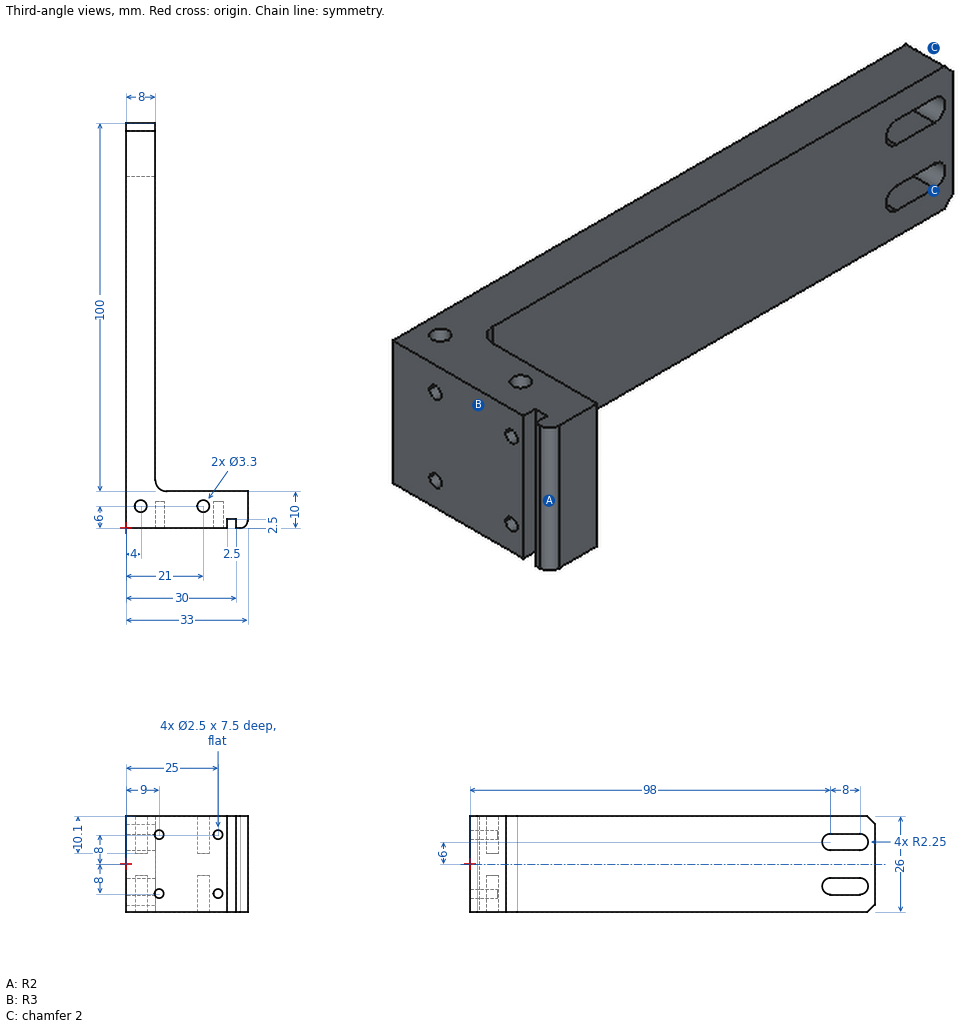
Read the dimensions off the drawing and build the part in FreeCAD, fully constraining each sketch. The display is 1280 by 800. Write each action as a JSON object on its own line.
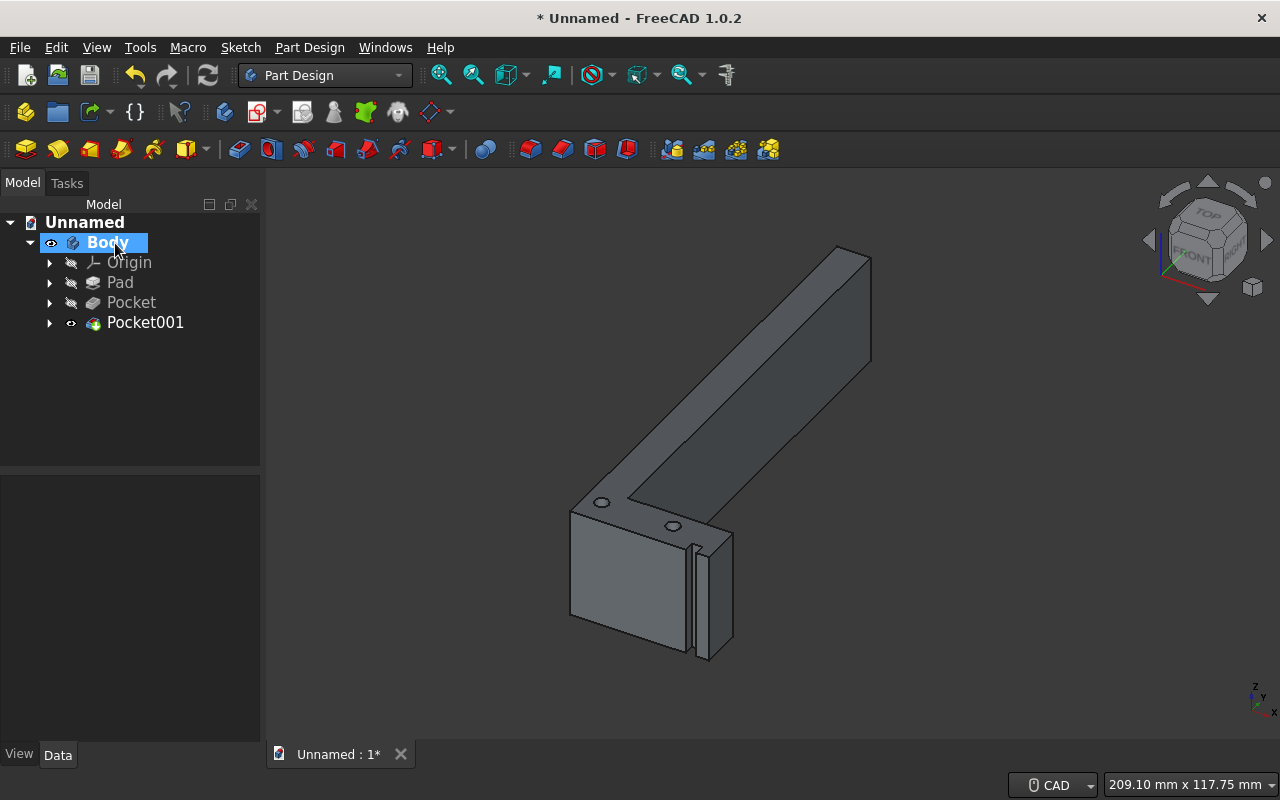
{"action": "left_click", "coordinate": [116, 323]}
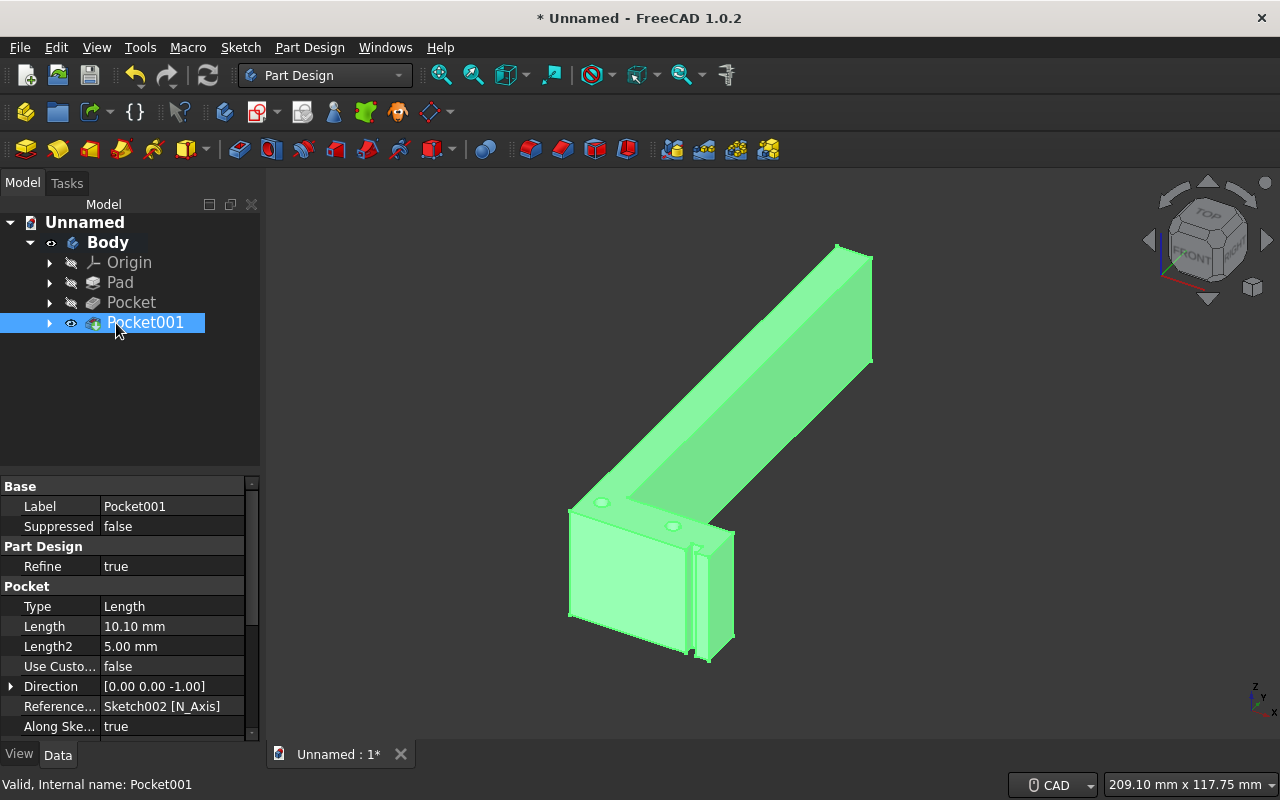
{"action": "left_click", "coordinate": [672, 150]}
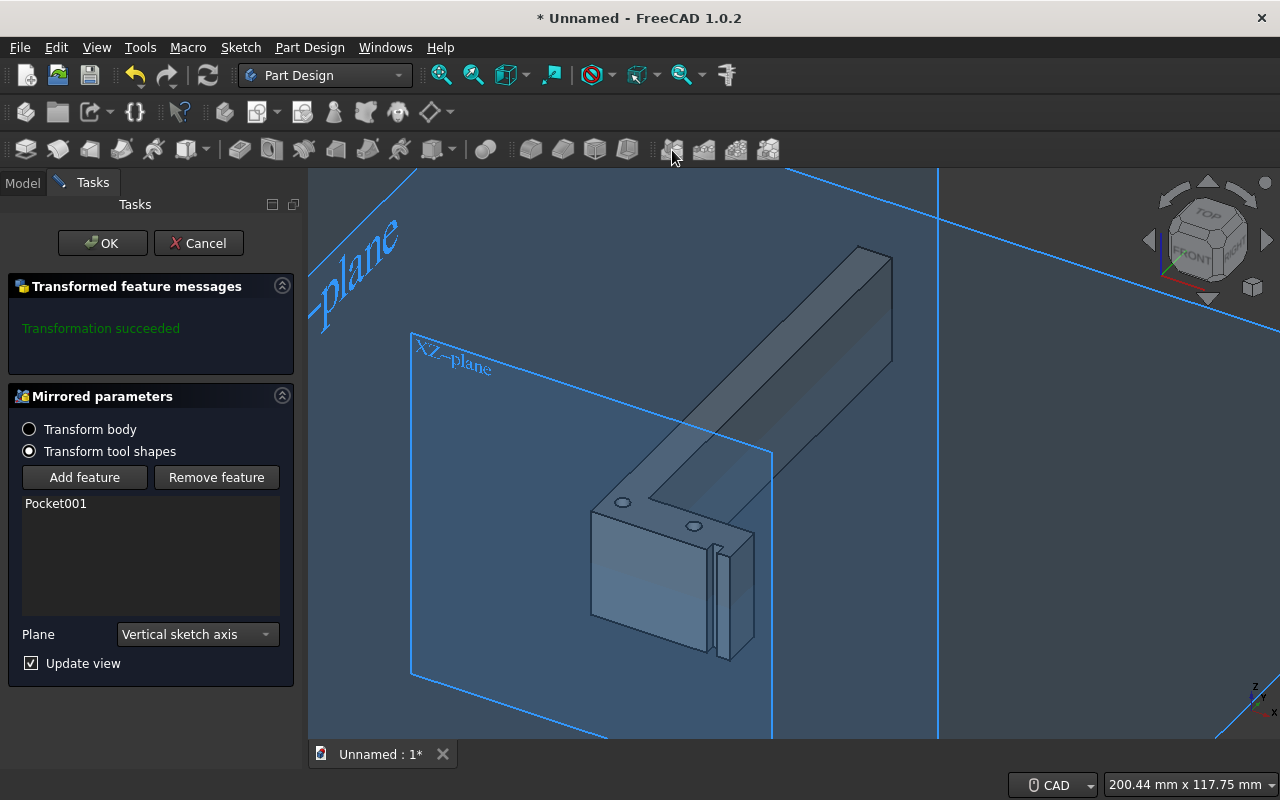
{"action": "left_click", "coordinate": [198, 634]}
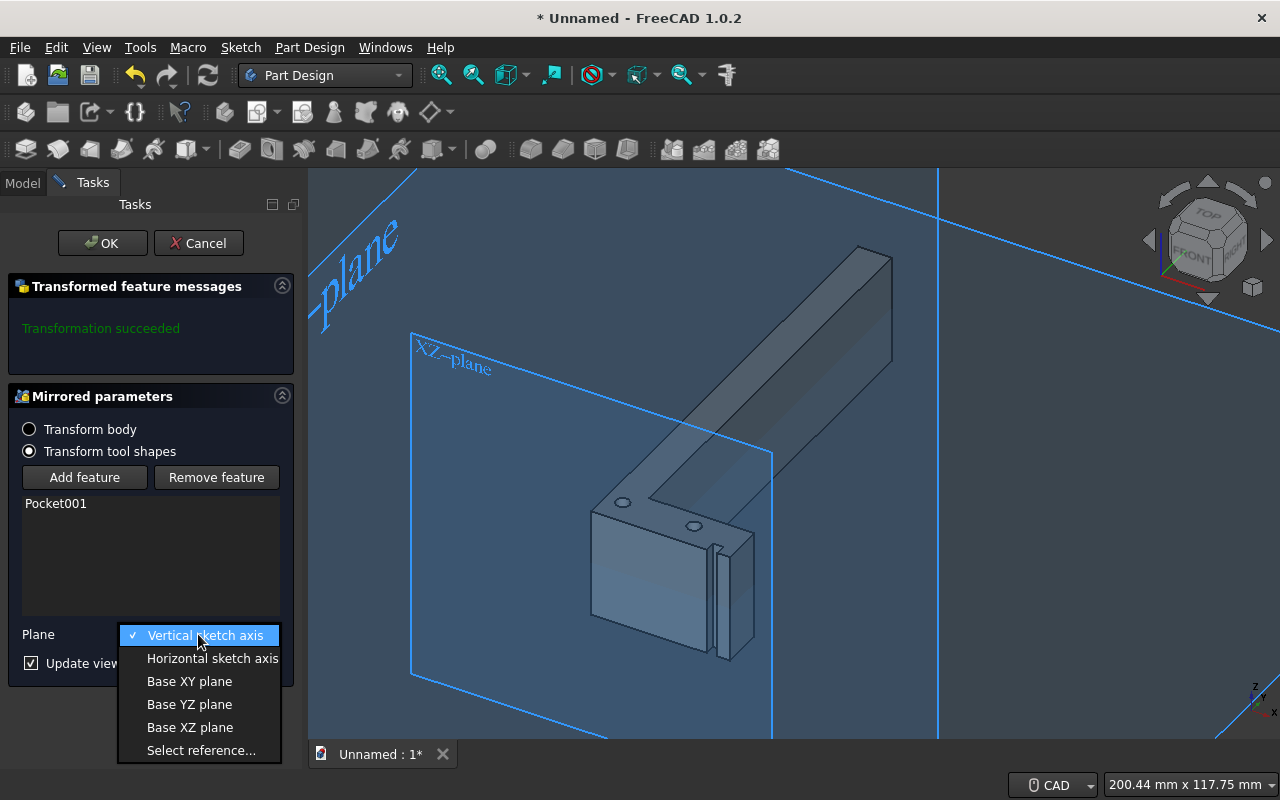
{"action": "left_click", "coordinate": [198, 682]}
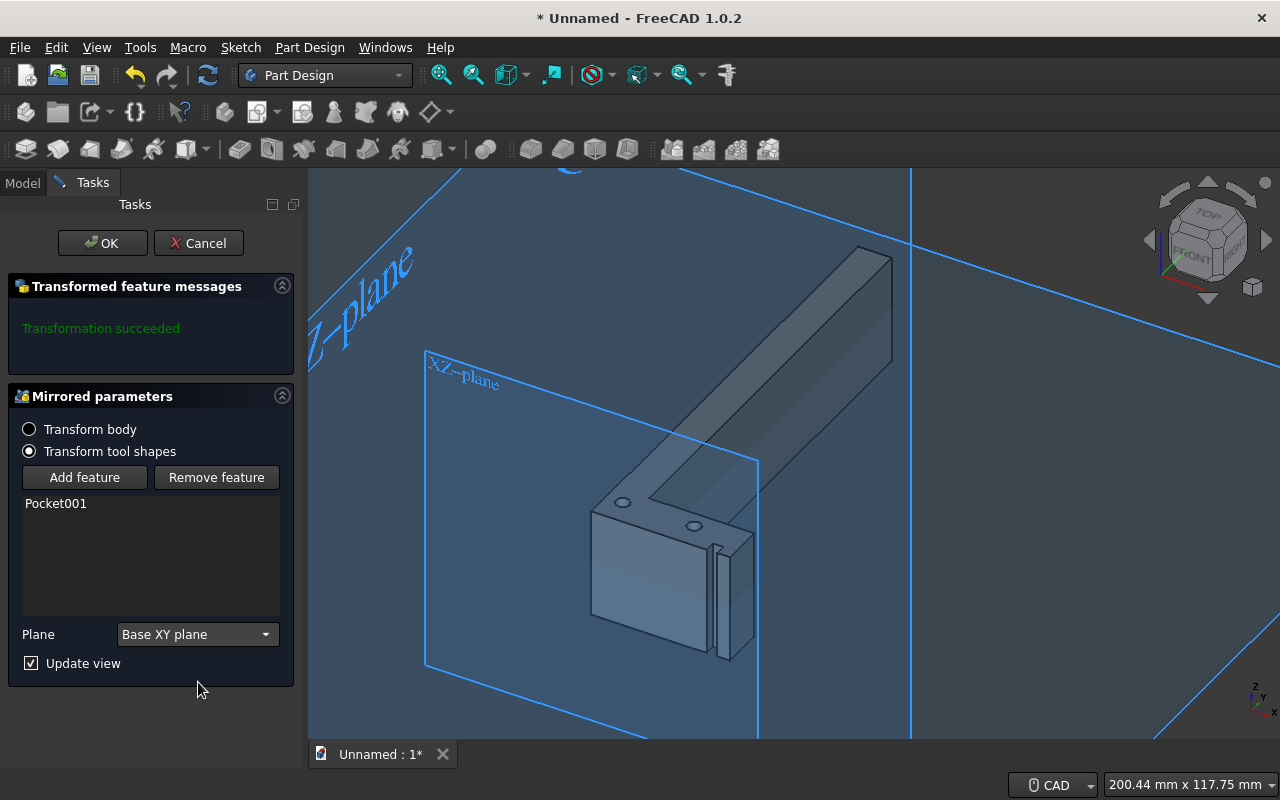
{"action": "left_click", "coordinate": [103, 243]}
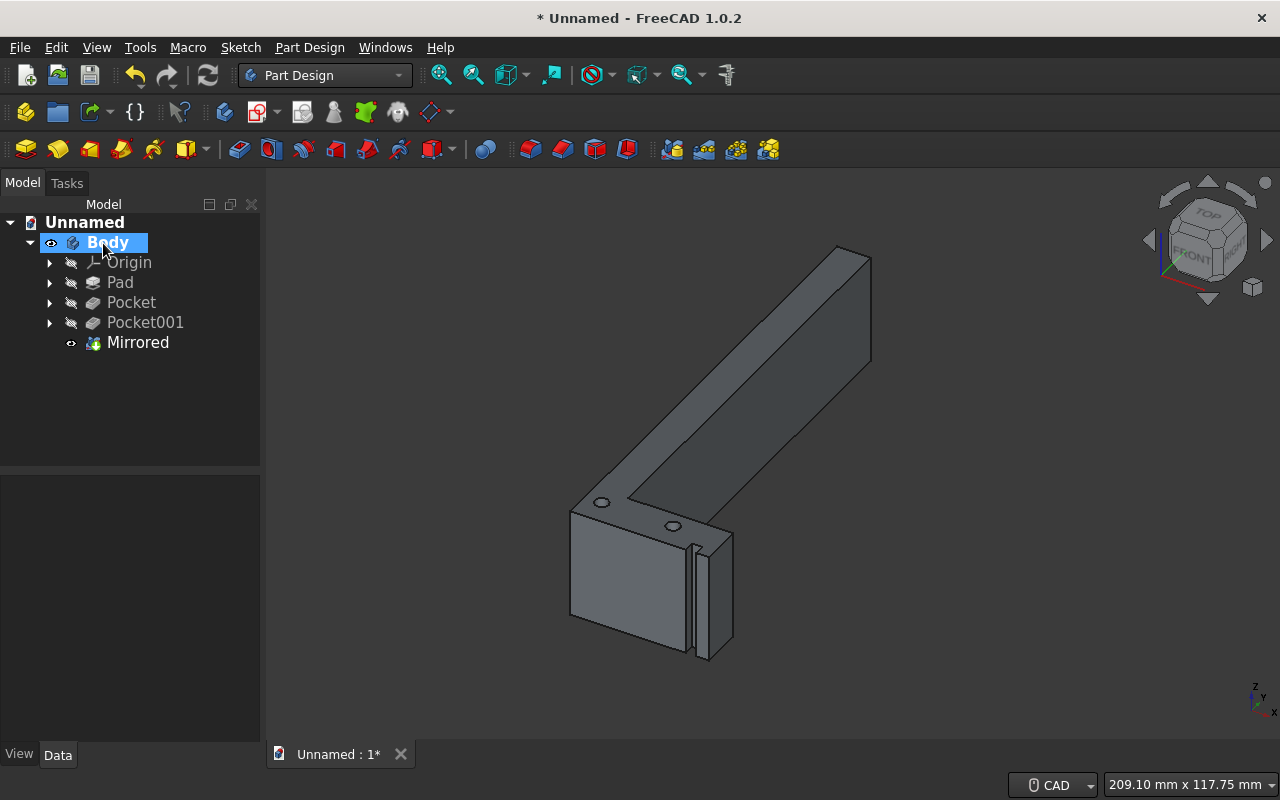
{"action": "left_click", "coordinate": [258, 112]}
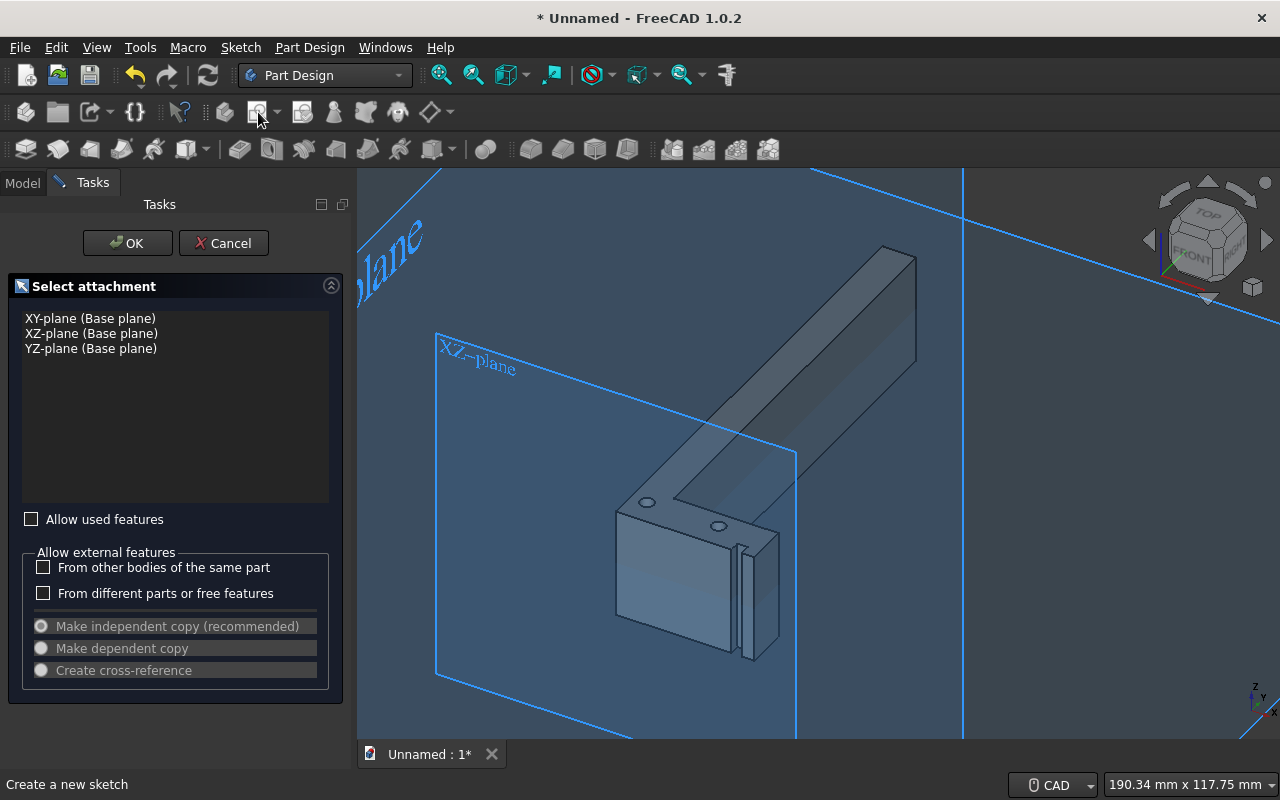
{"action": "left_click", "coordinate": [82, 334]}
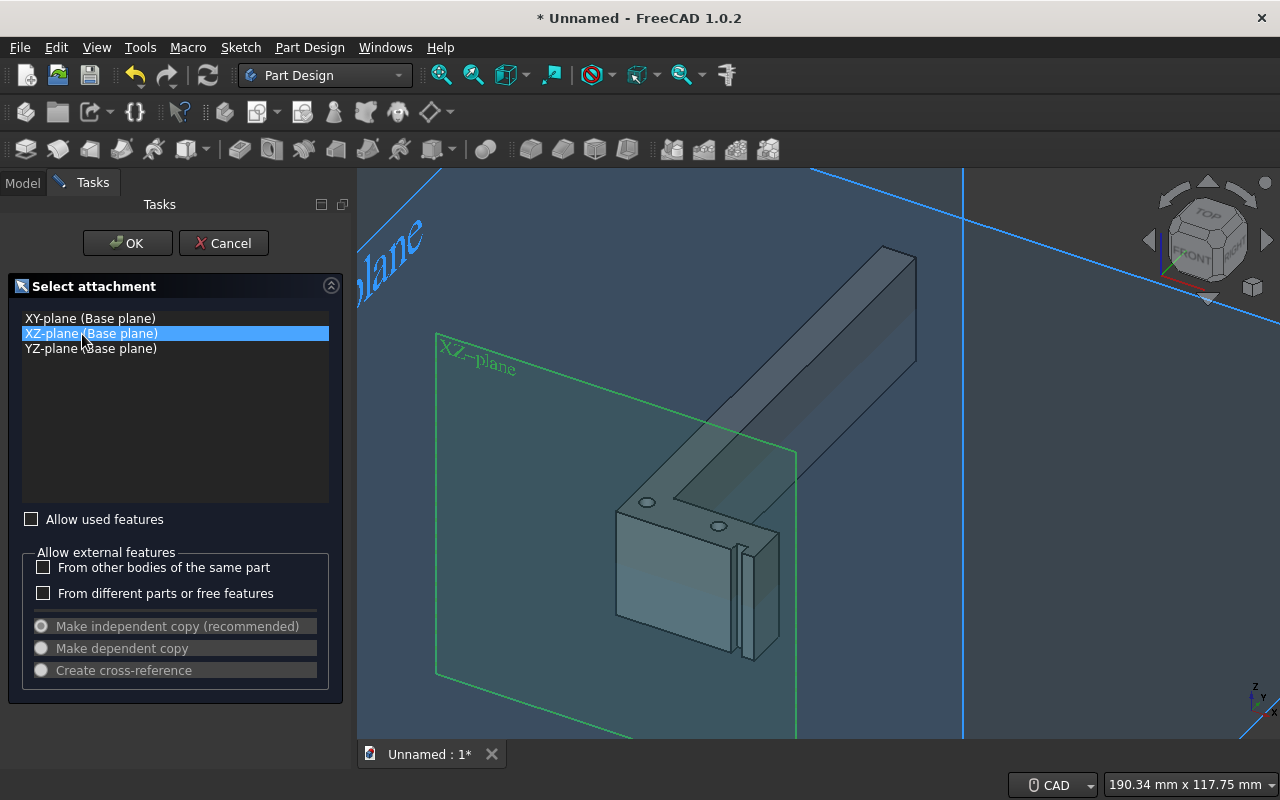
{"action": "left_click", "coordinate": [128, 243]}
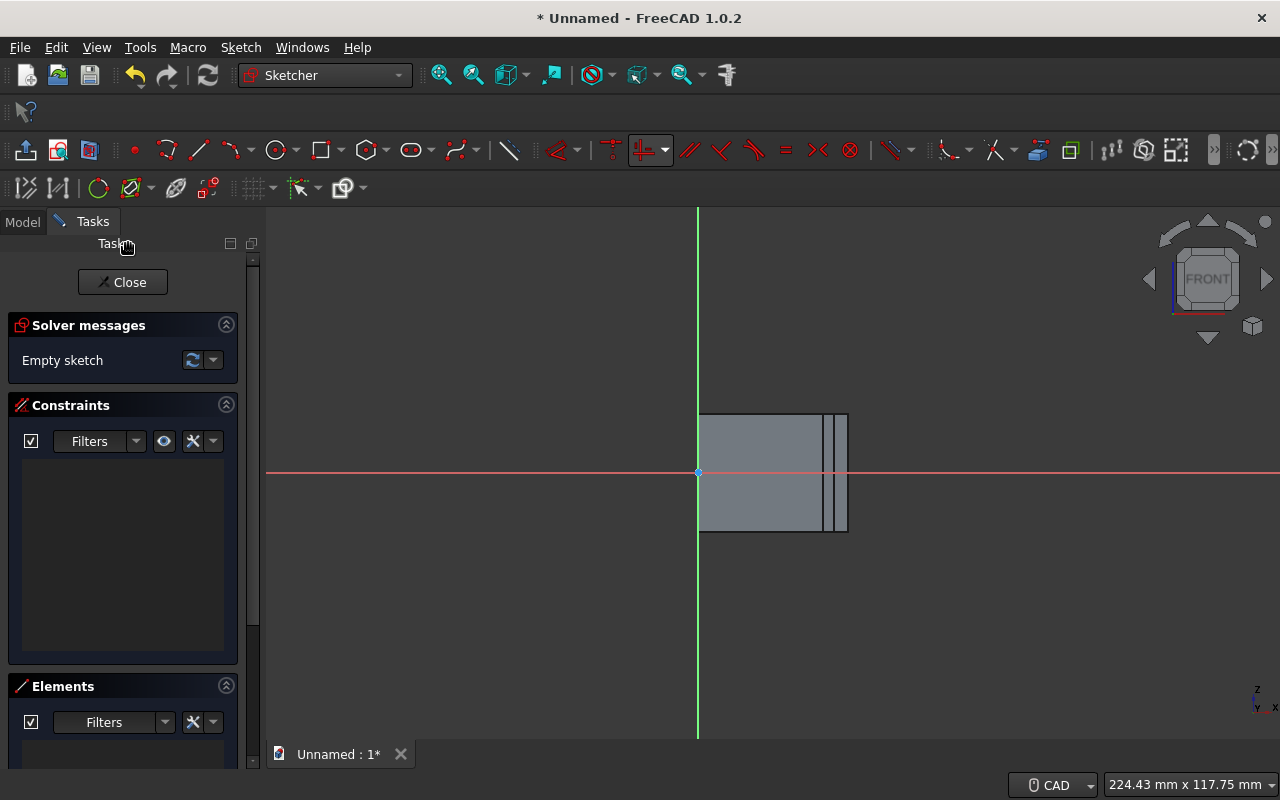
{"action": "scroll", "coordinate": [775, 473], "scroll_direction": "up", "scroll_amount": 7}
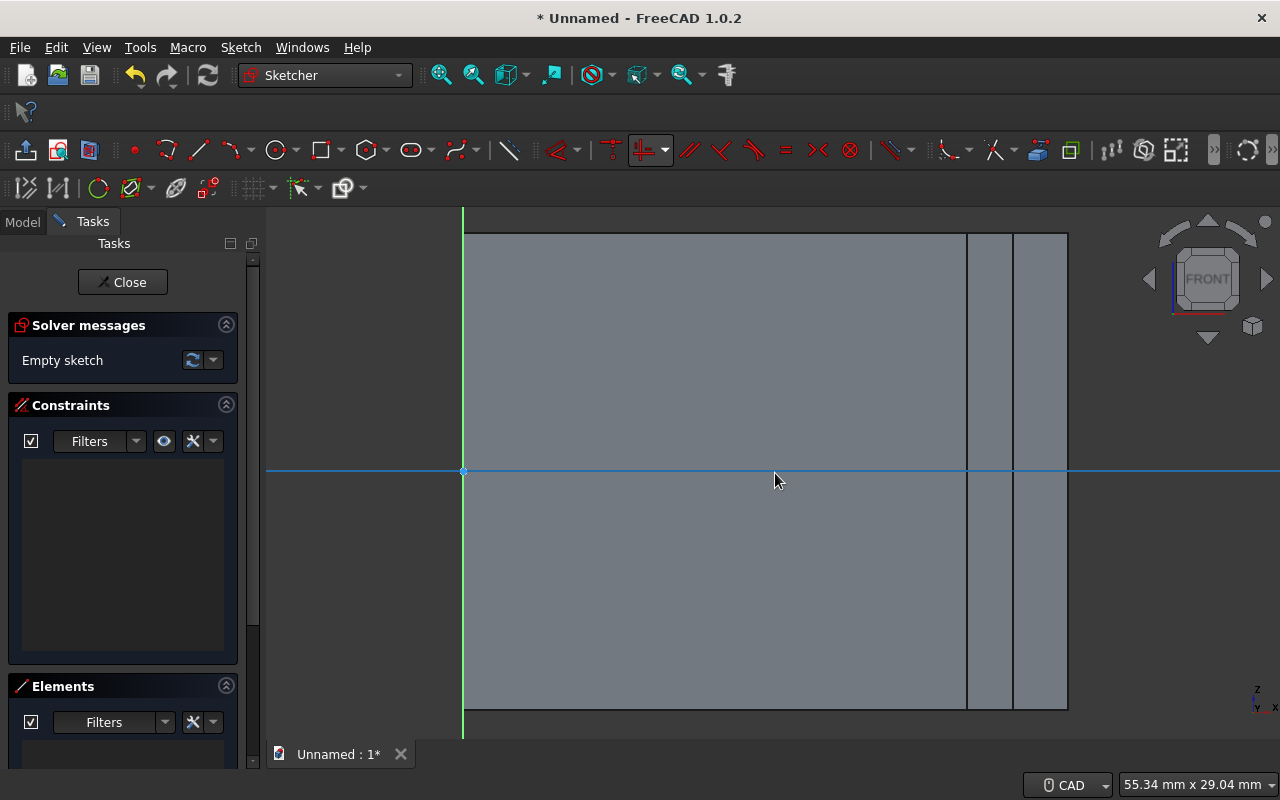
{"action": "left_click", "coordinate": [276, 150]}